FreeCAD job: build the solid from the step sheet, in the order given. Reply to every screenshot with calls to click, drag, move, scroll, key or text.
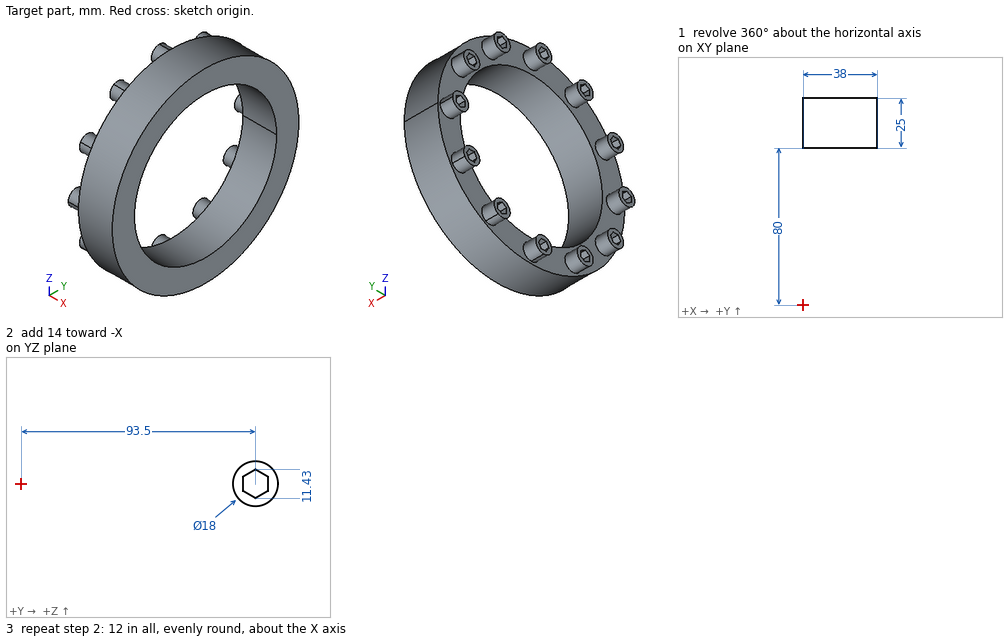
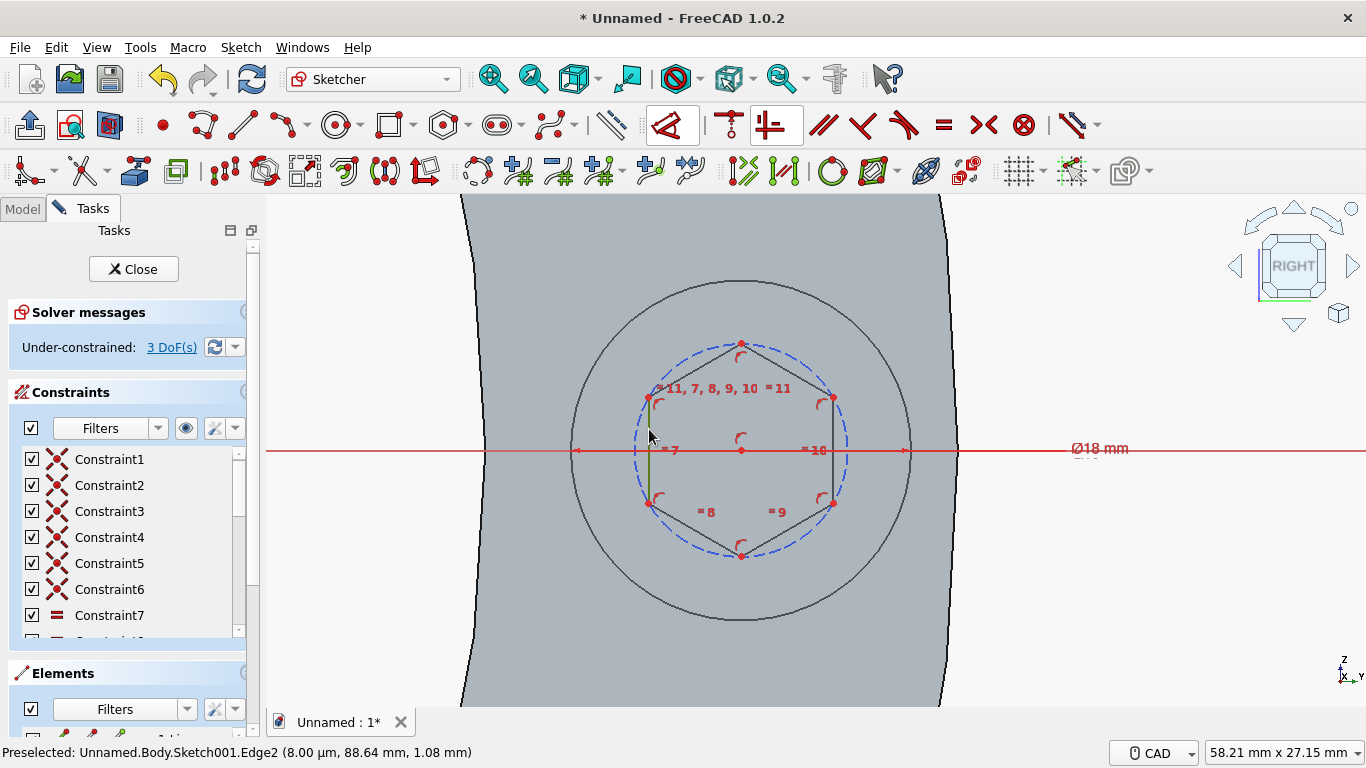
key(v)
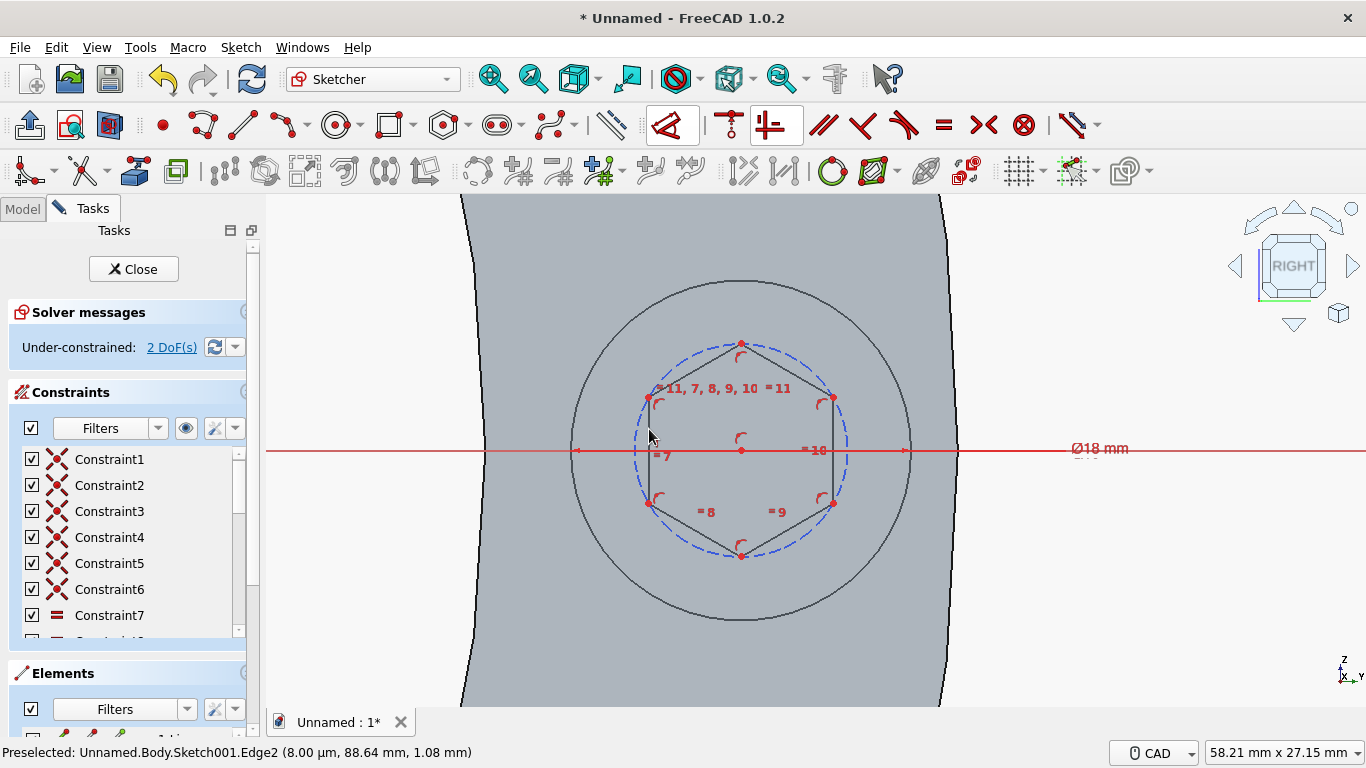
key(d)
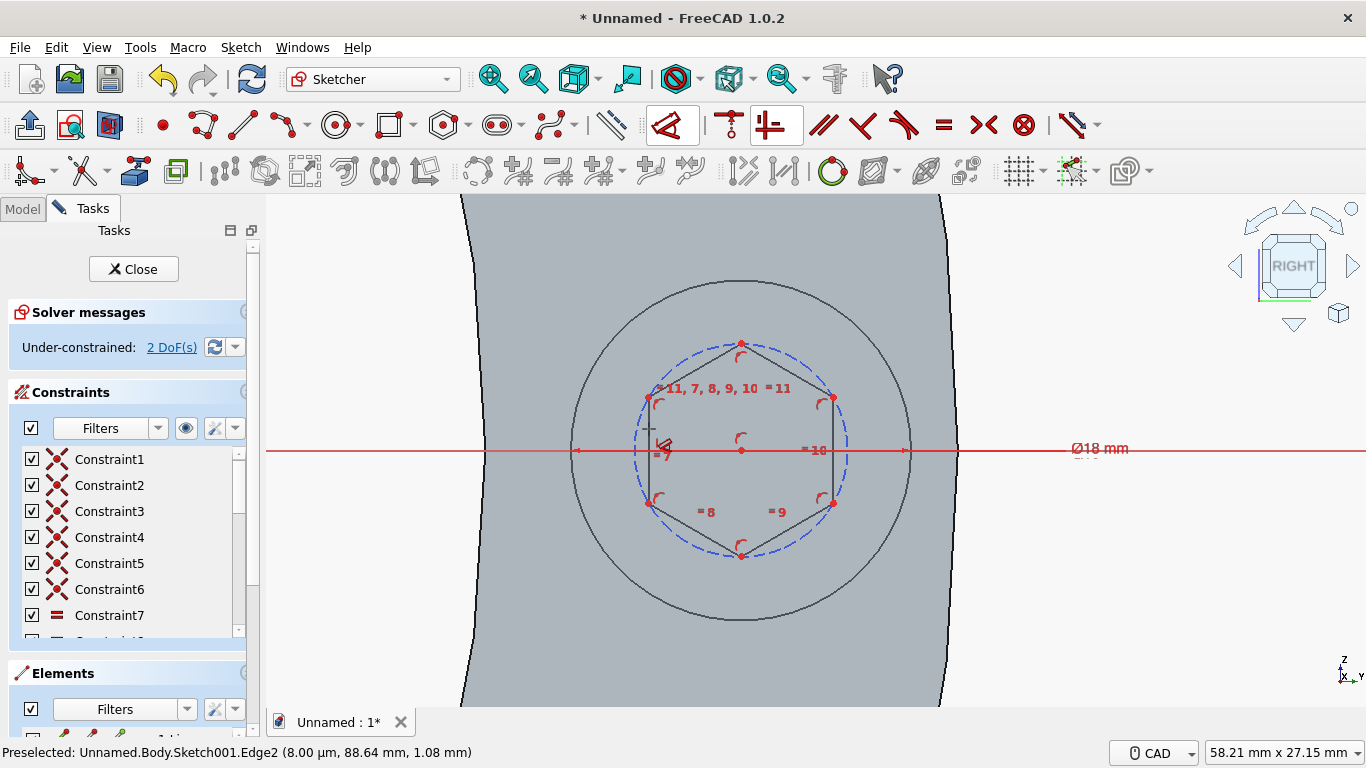
click(741, 557)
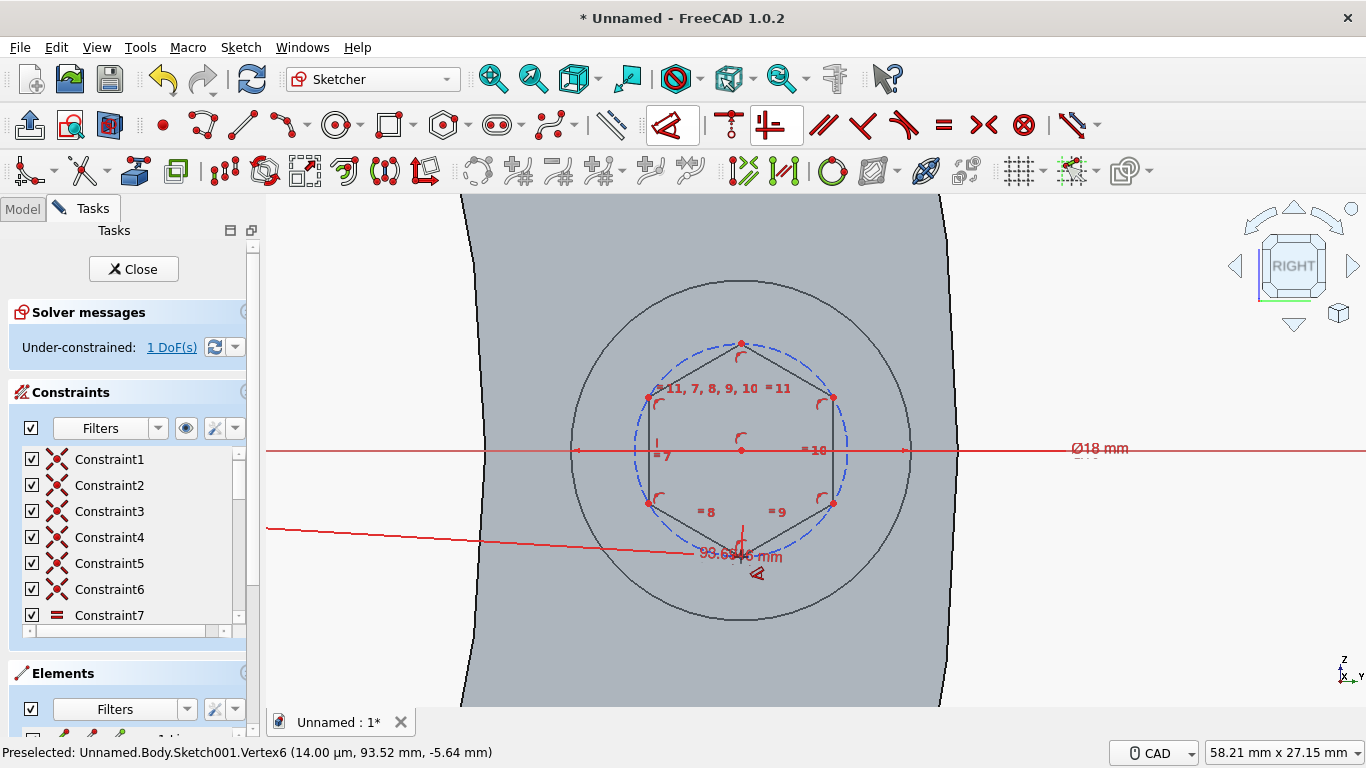
click(741, 344)
click(775, 402)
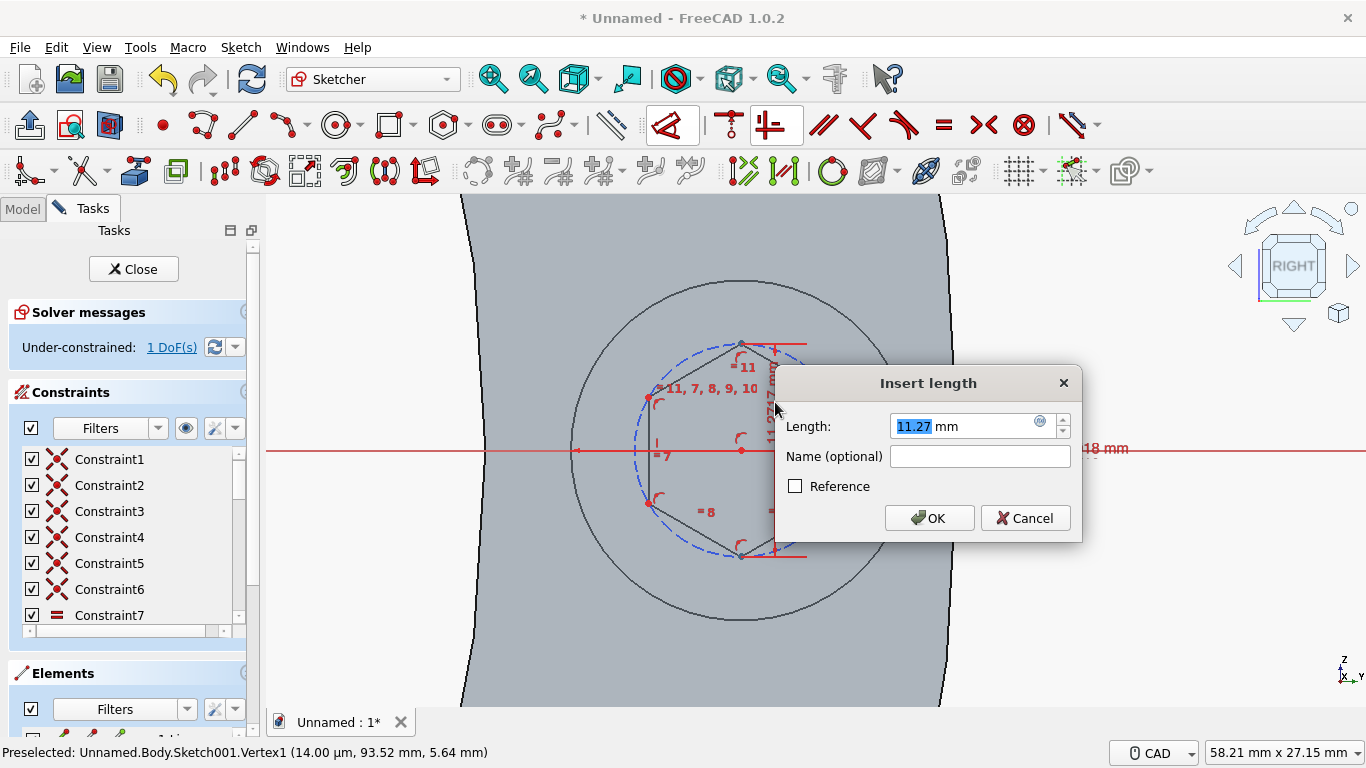
text(11.43)
key(Return)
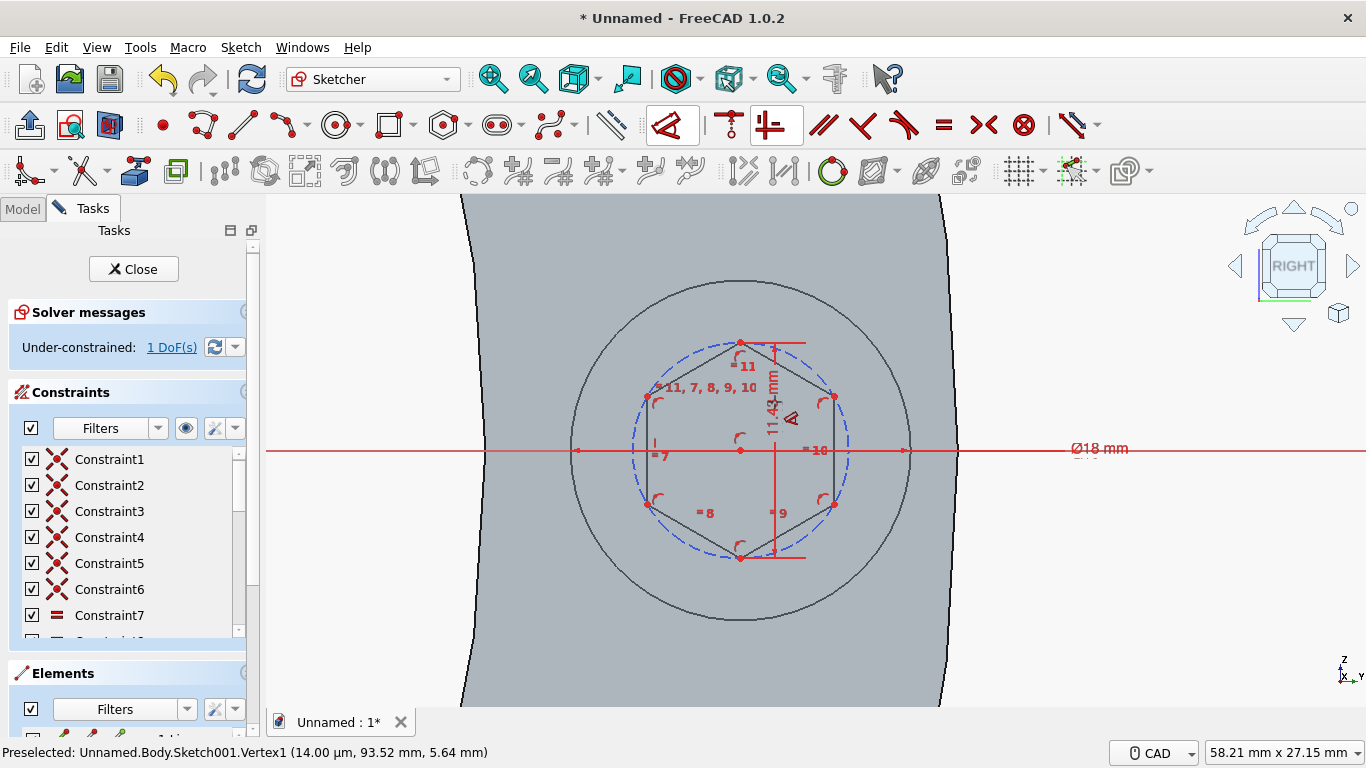
click(741, 450)
click(517, 484)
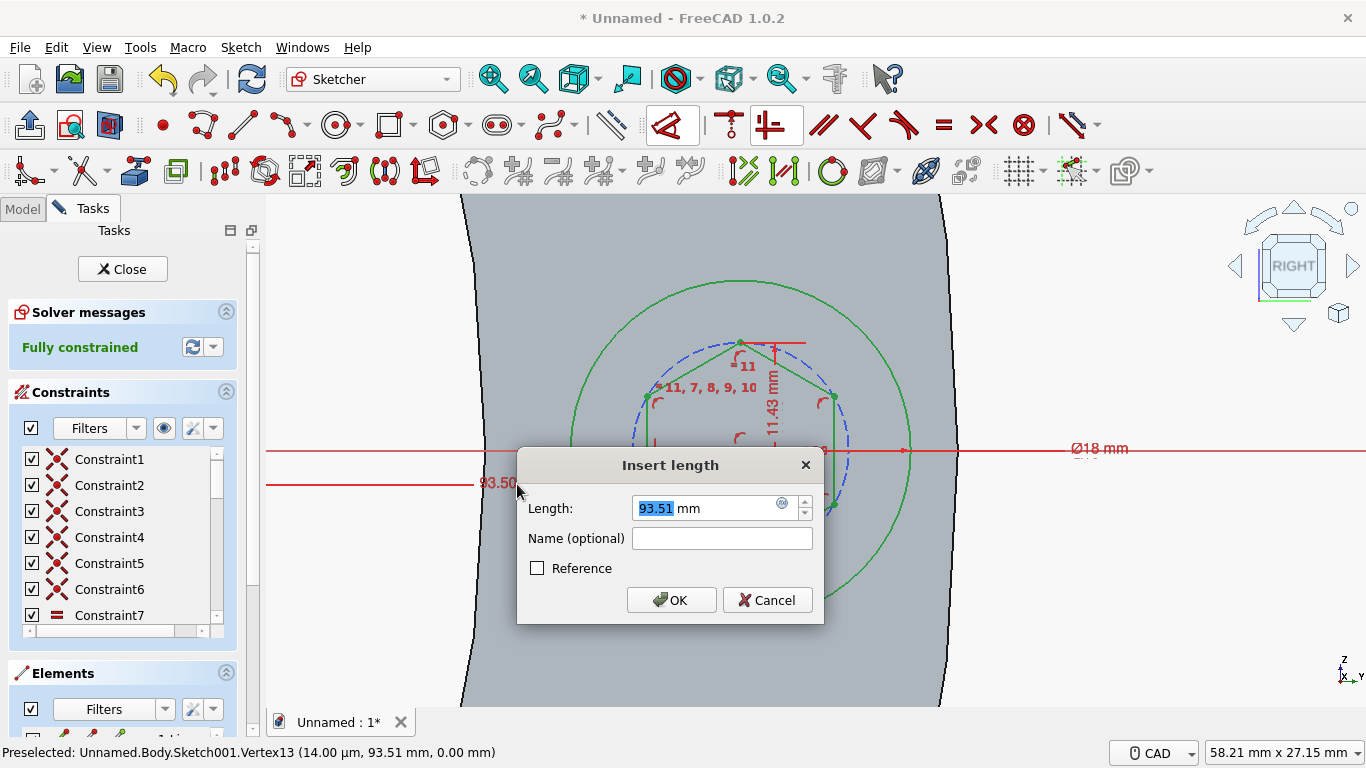
text(93.5)
key(Return)
key(Escape)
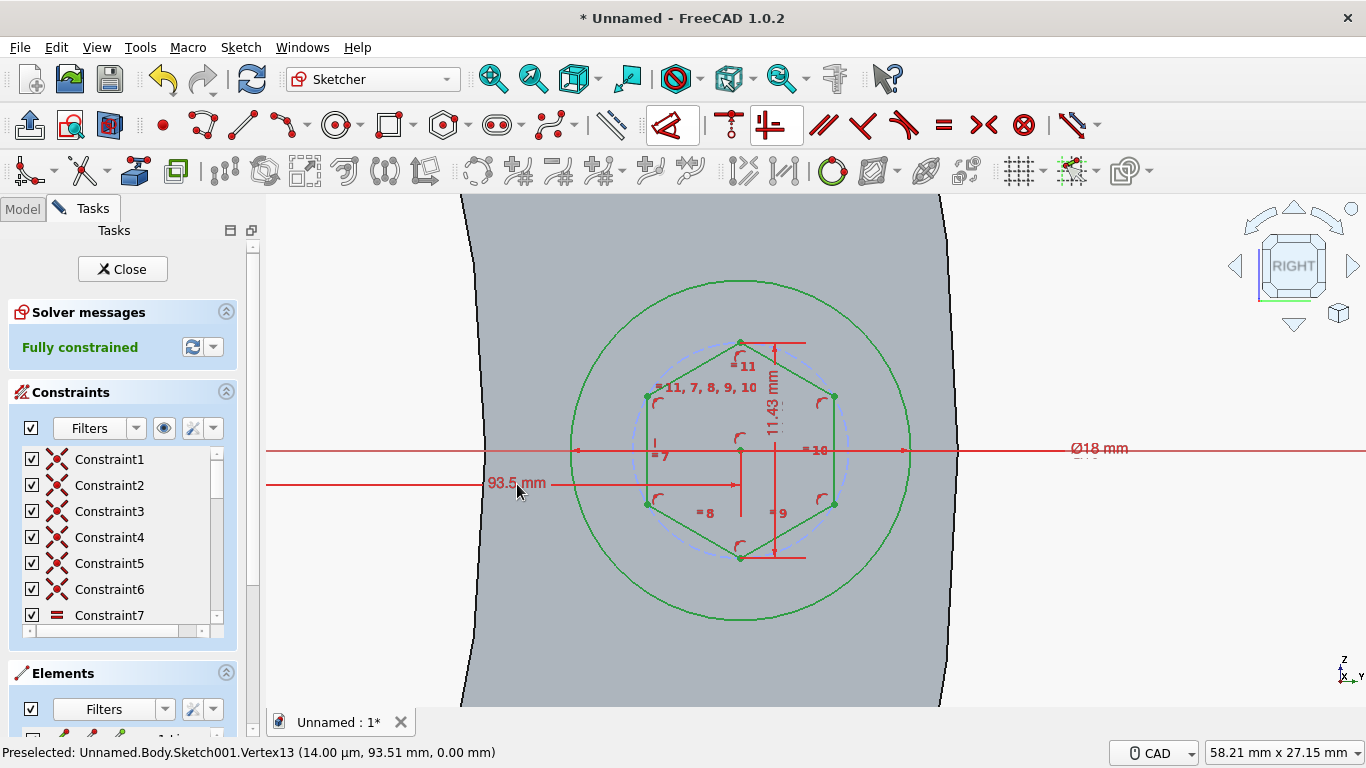
click(123, 269)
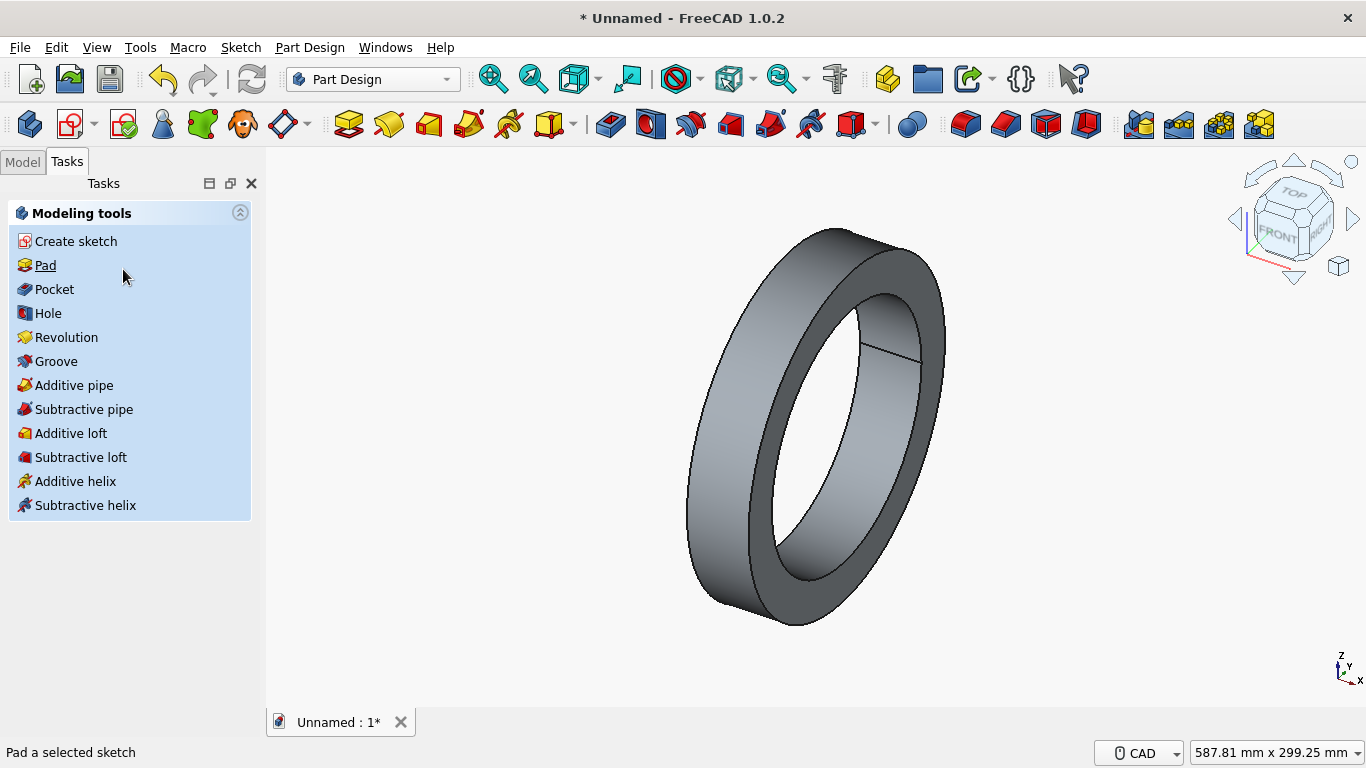
click(350, 124)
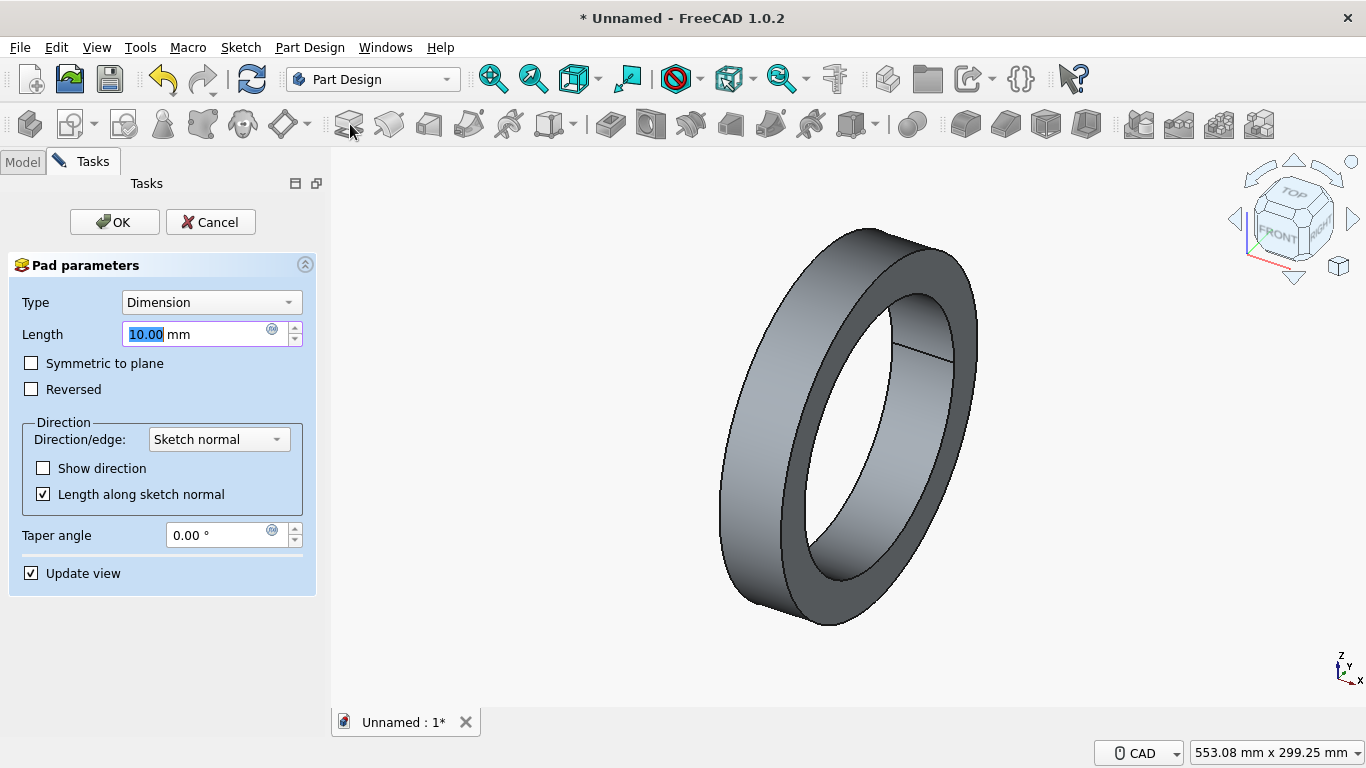
text(14)
key(Tab)